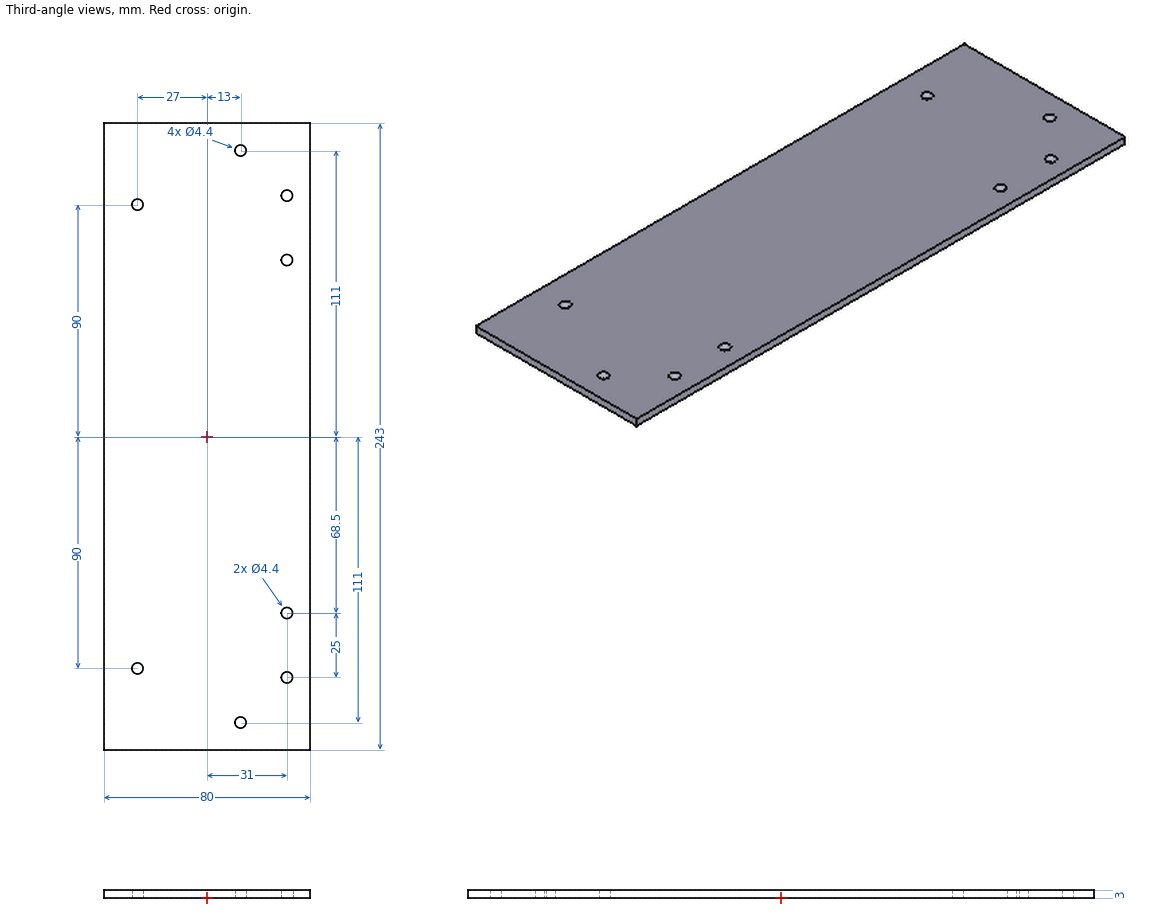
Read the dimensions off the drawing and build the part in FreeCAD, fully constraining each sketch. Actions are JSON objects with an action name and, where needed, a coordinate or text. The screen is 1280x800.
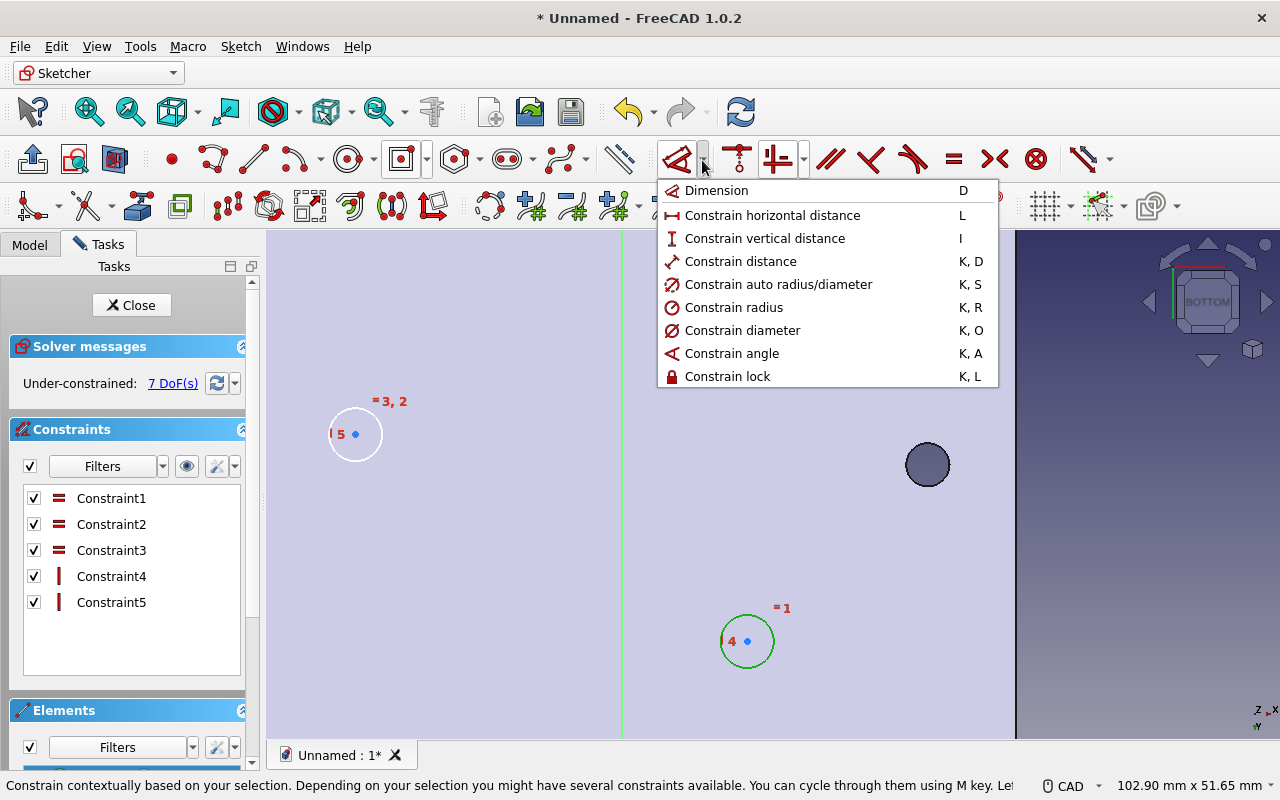
{"action": "left_click", "coordinate": [828, 330]}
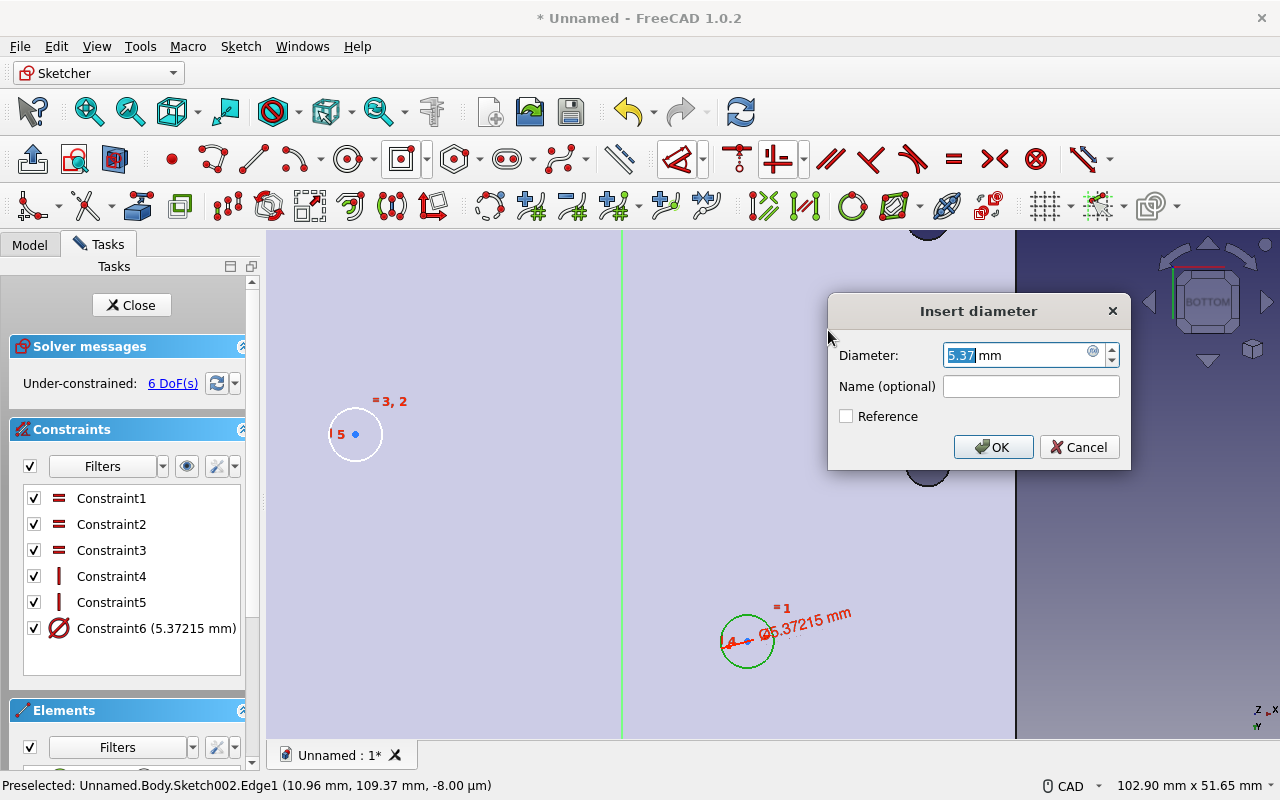
{"action": "type", "text": "4.4"}
{"action": "key", "text": "Return"}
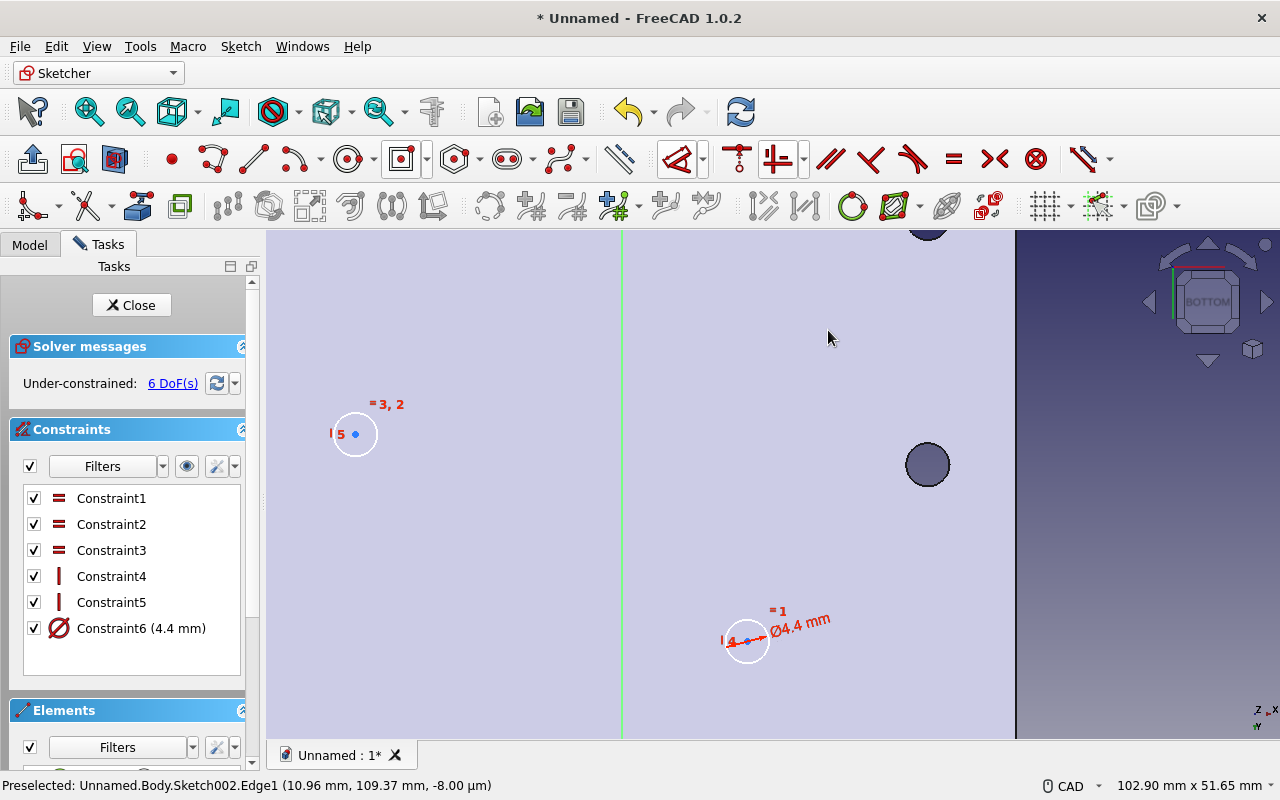
{"action": "scroll", "coordinate": [728, 632], "scroll_direction": "down", "scroll_amount": 10}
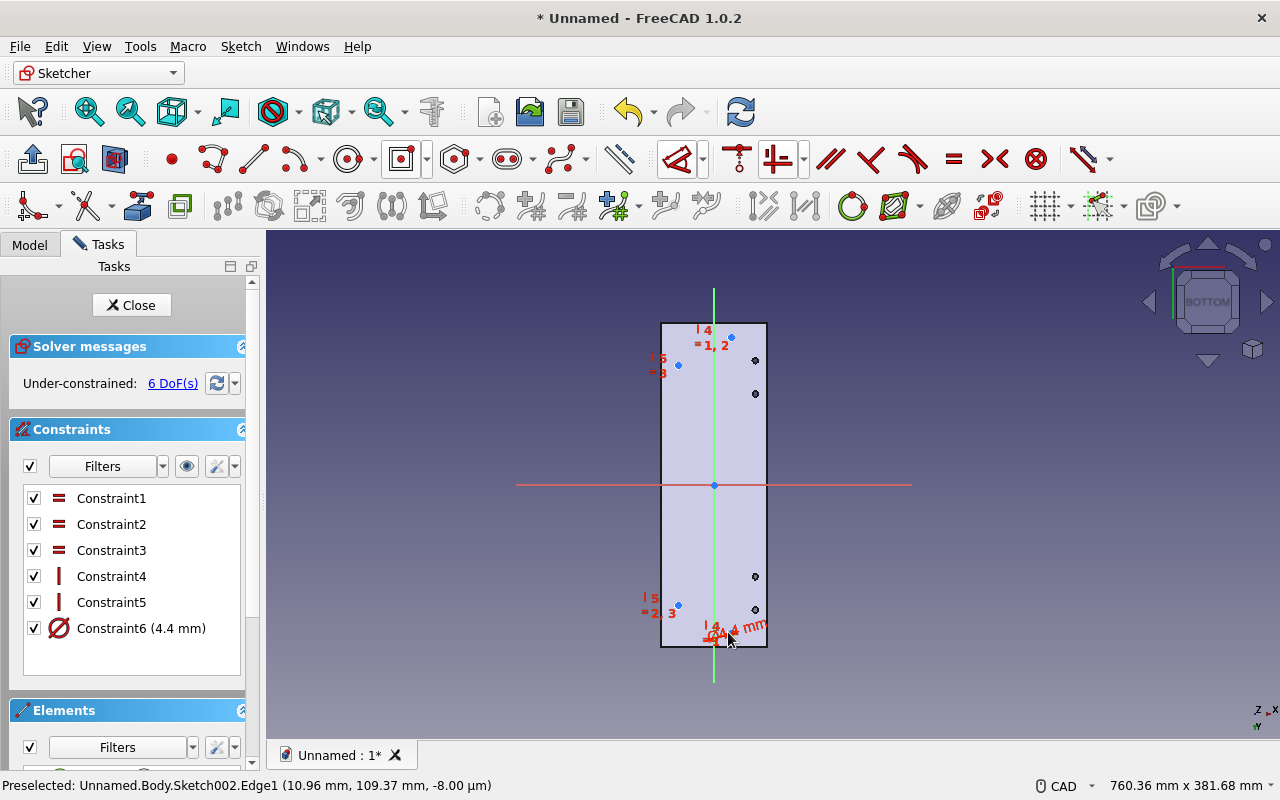
{"action": "scroll", "coordinate": [731, 634], "scroll_direction": "up", "scroll_amount": 5}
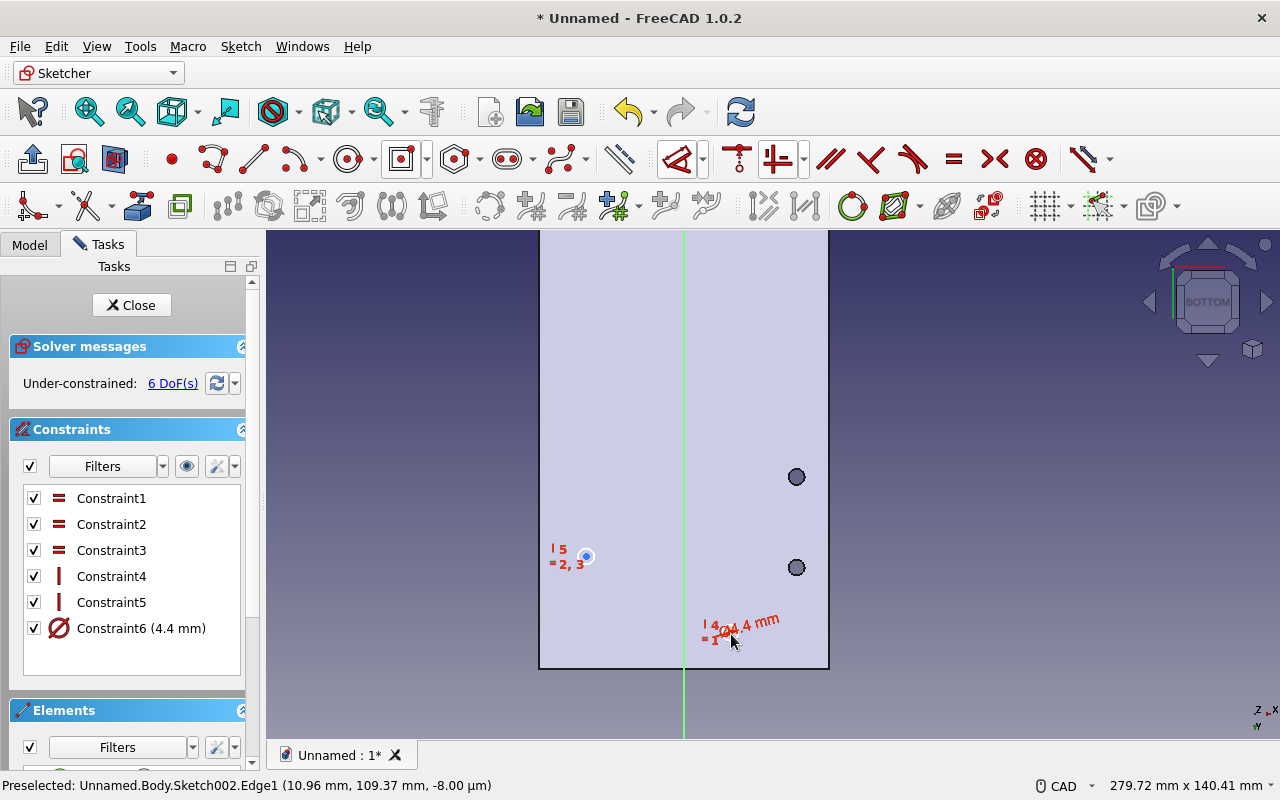
{"action": "left_click", "coordinate": [730, 633]}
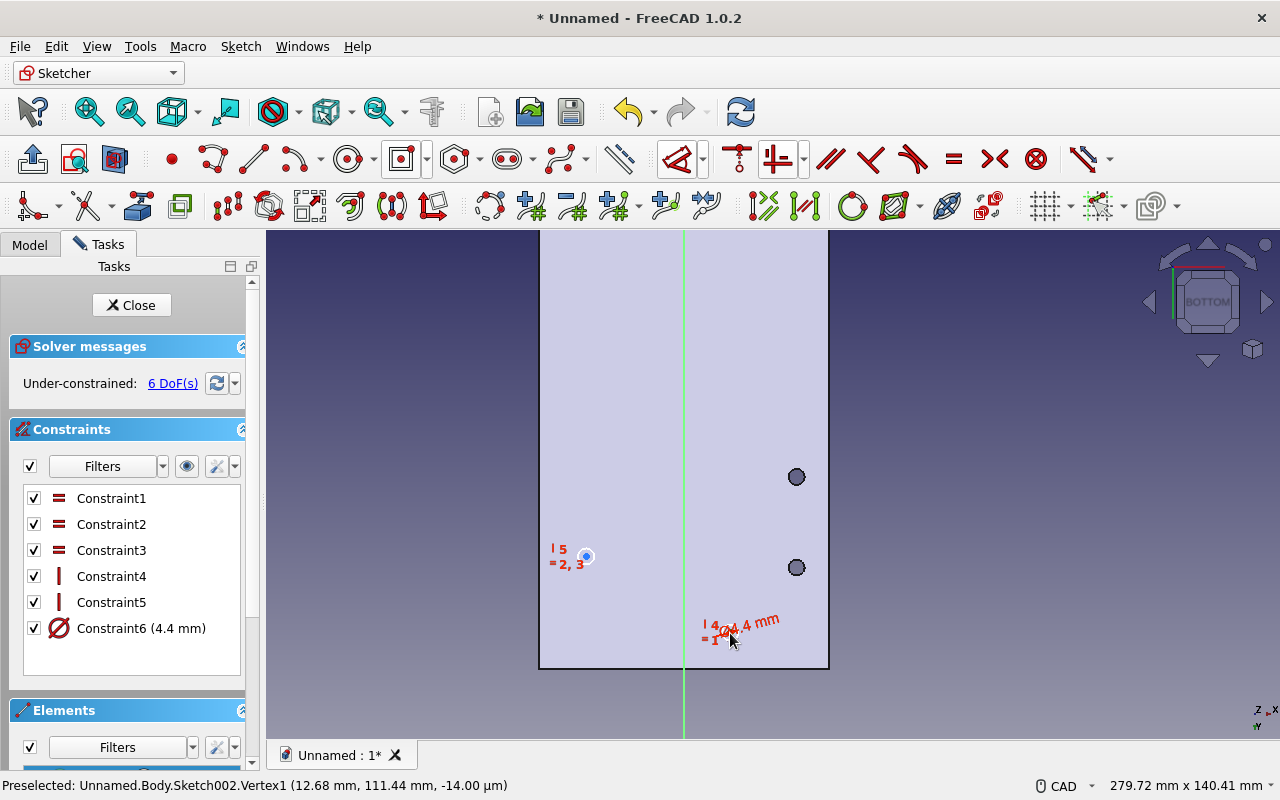
{"action": "key", "text": "l"}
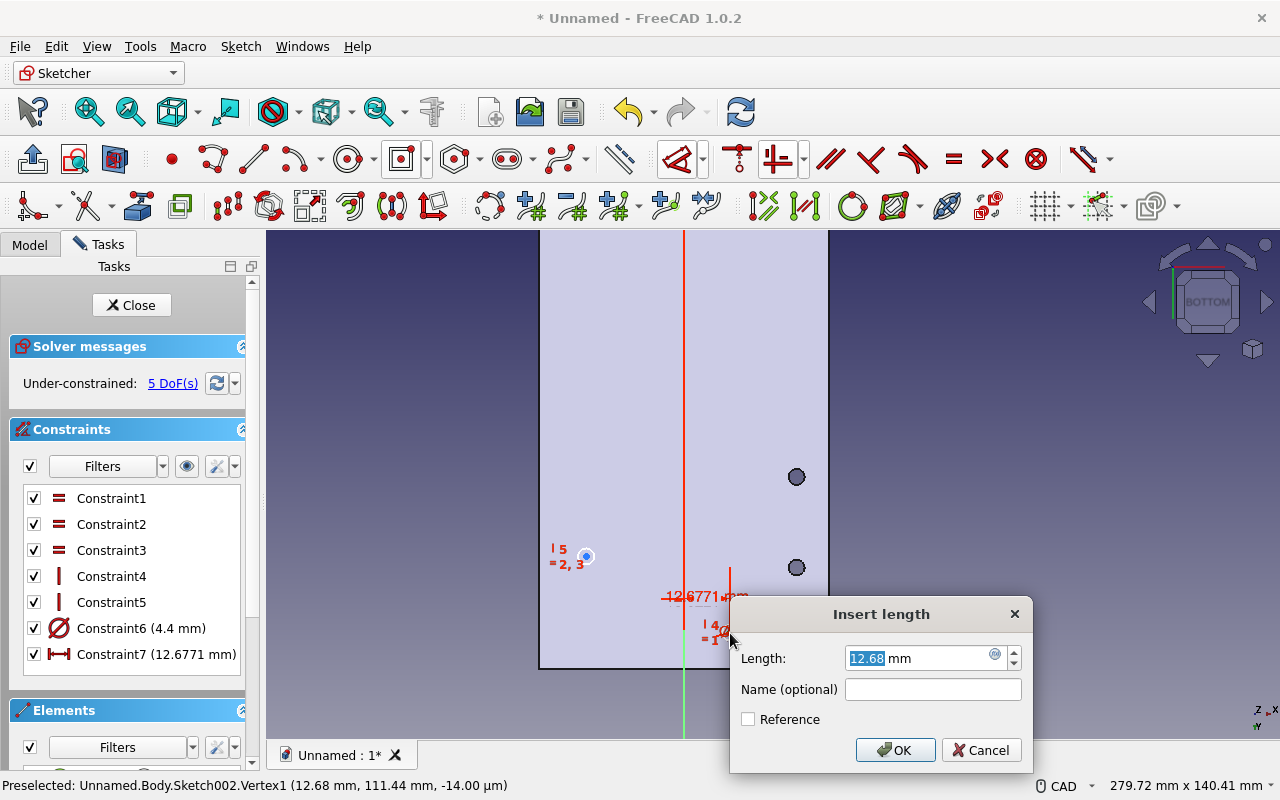
{"action": "type", "text": "13"}
{"action": "key", "text": "Return"}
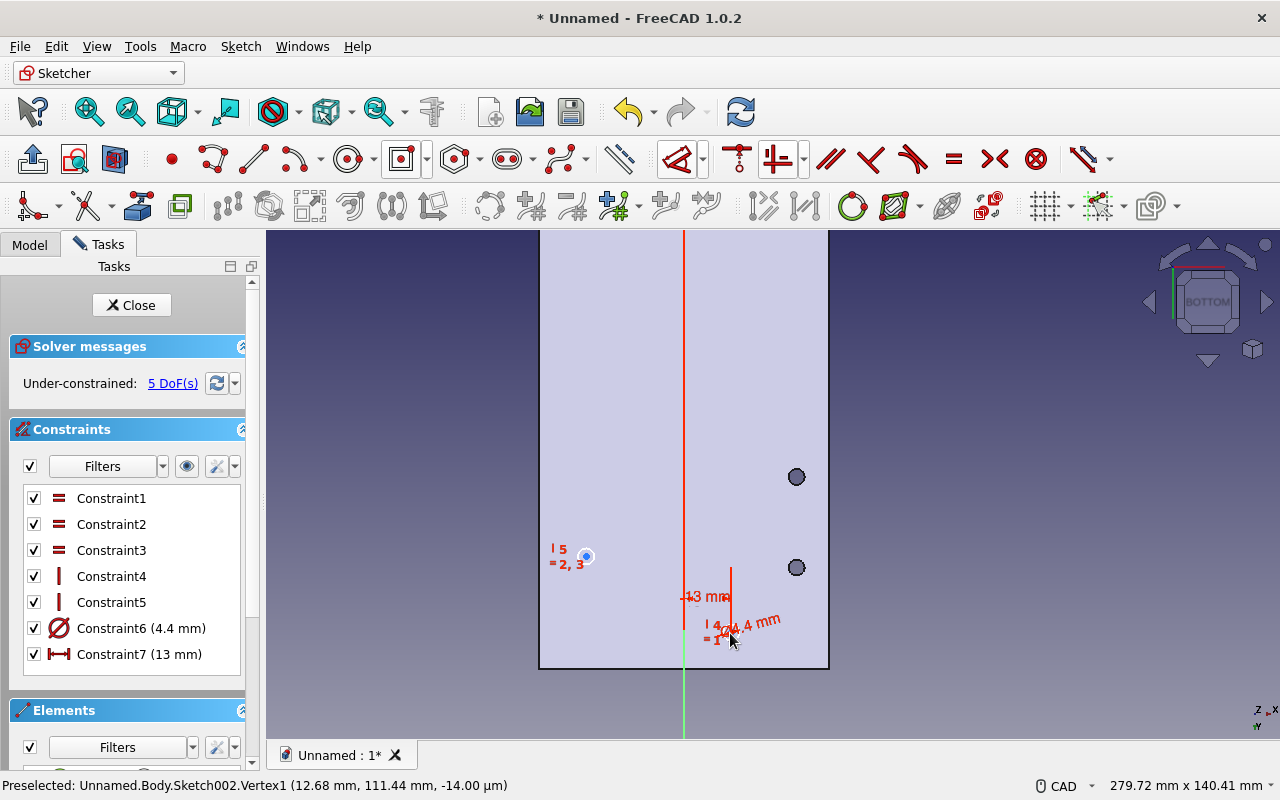
{"action": "left_click", "coordinate": [586, 556]}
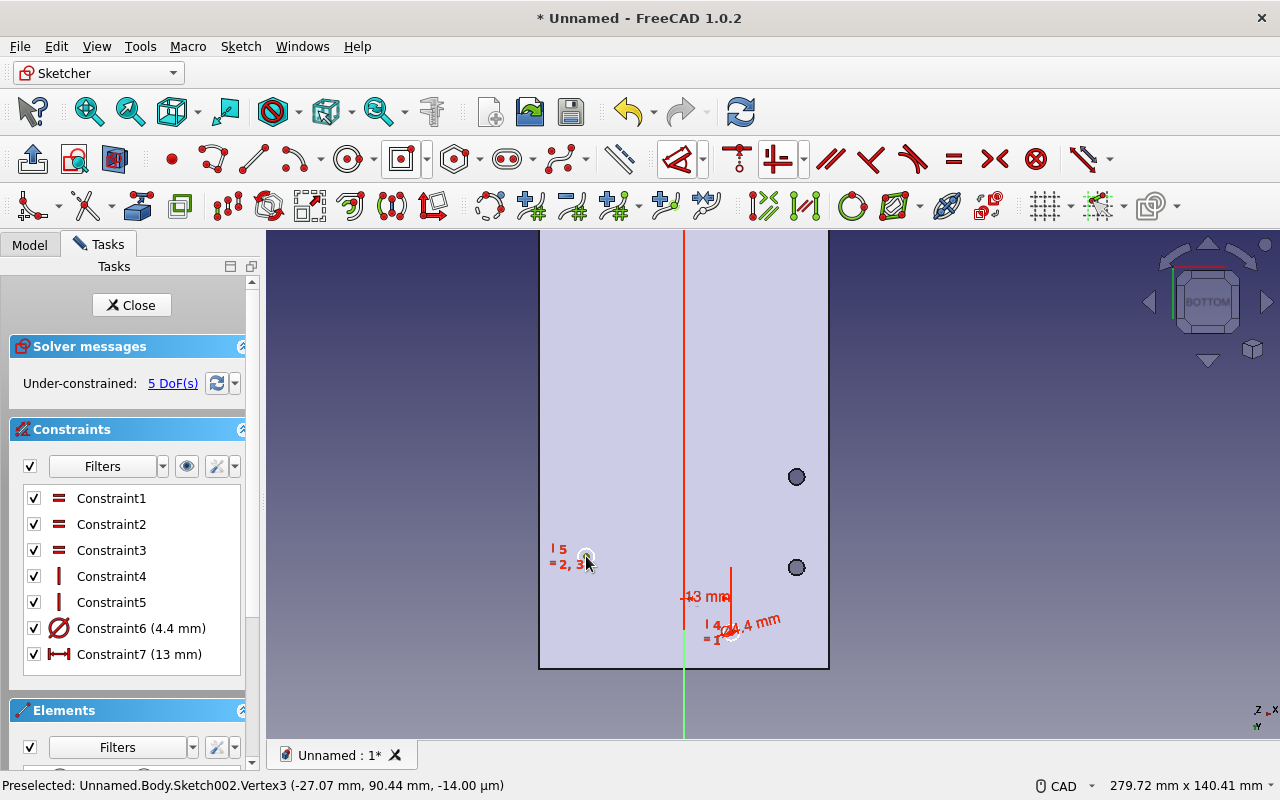
{"action": "left_click", "coordinate": [702, 160]}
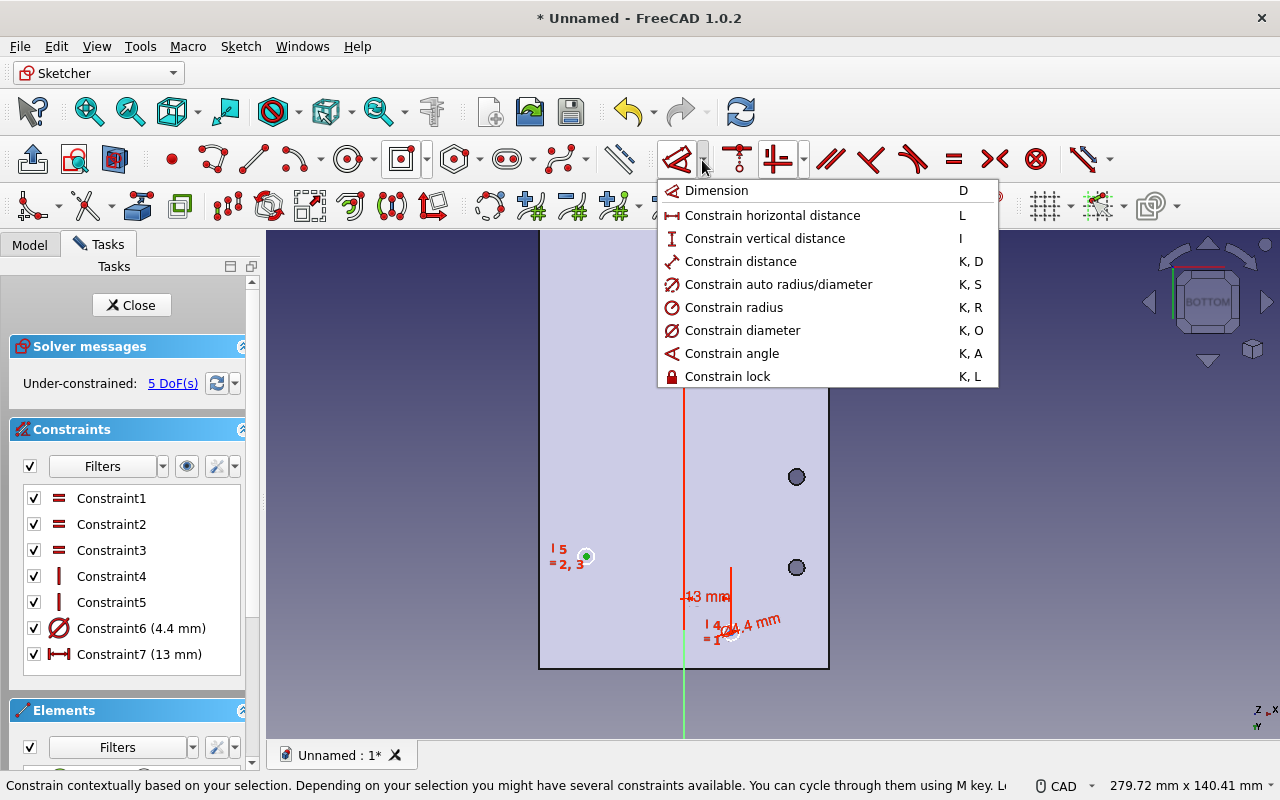
{"action": "left_click", "coordinate": [828, 216]}